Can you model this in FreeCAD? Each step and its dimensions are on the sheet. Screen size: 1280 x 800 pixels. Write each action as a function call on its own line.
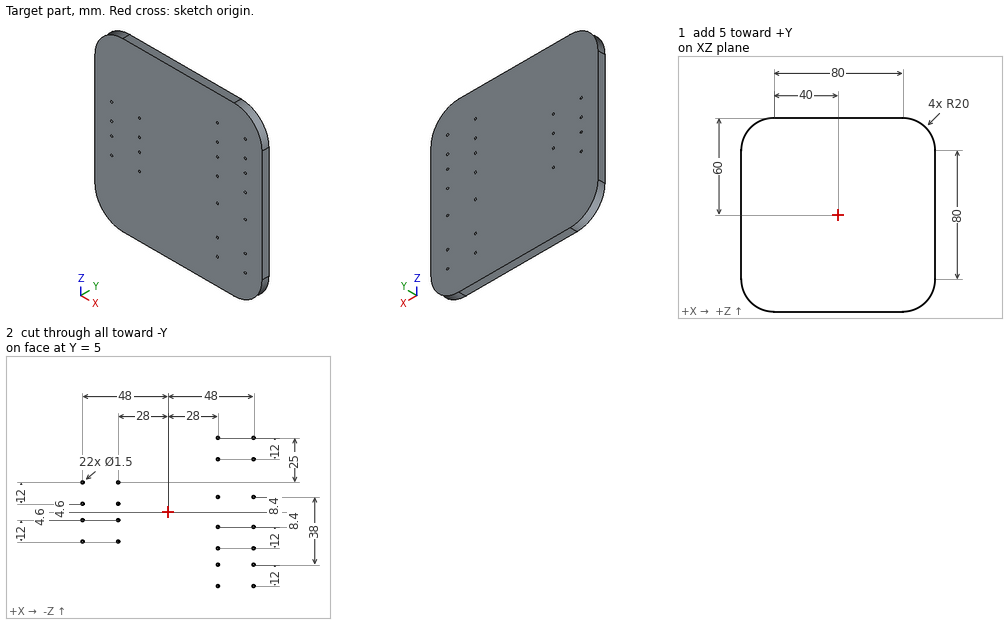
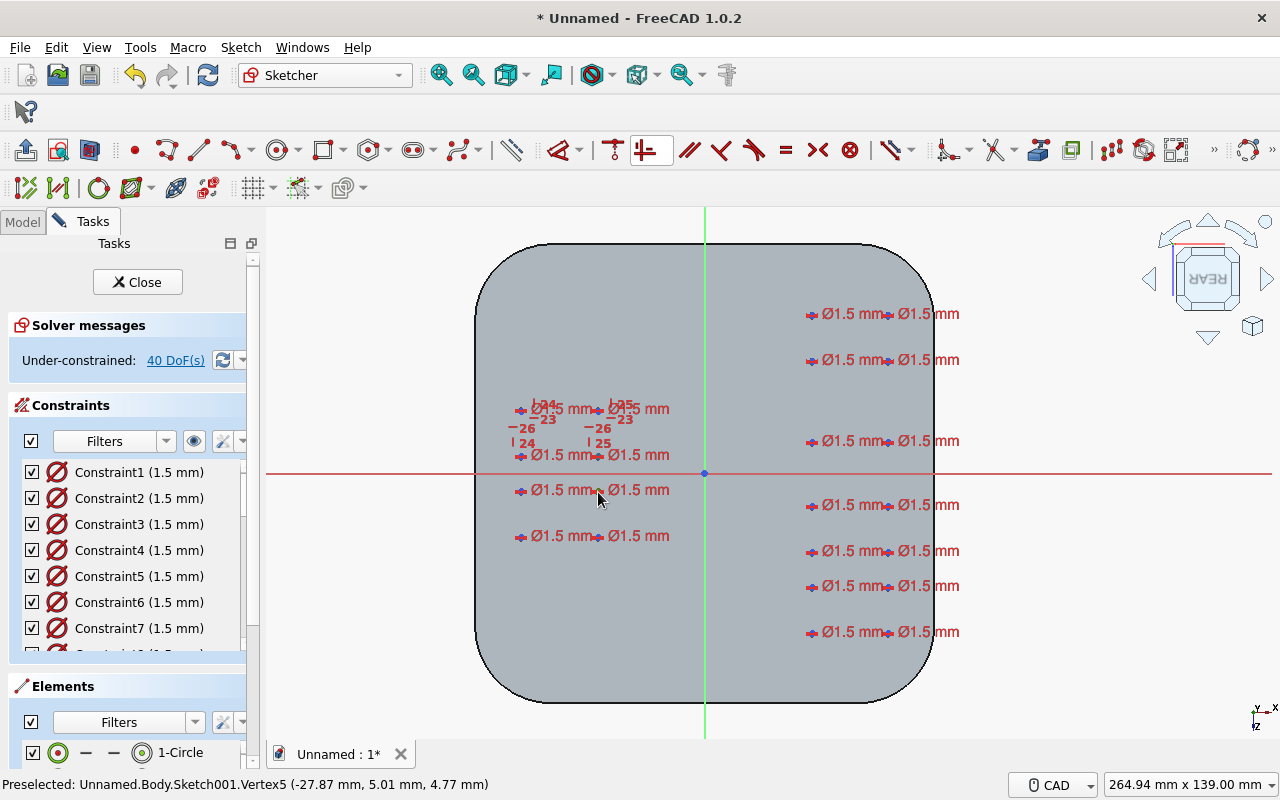
click(668, 150)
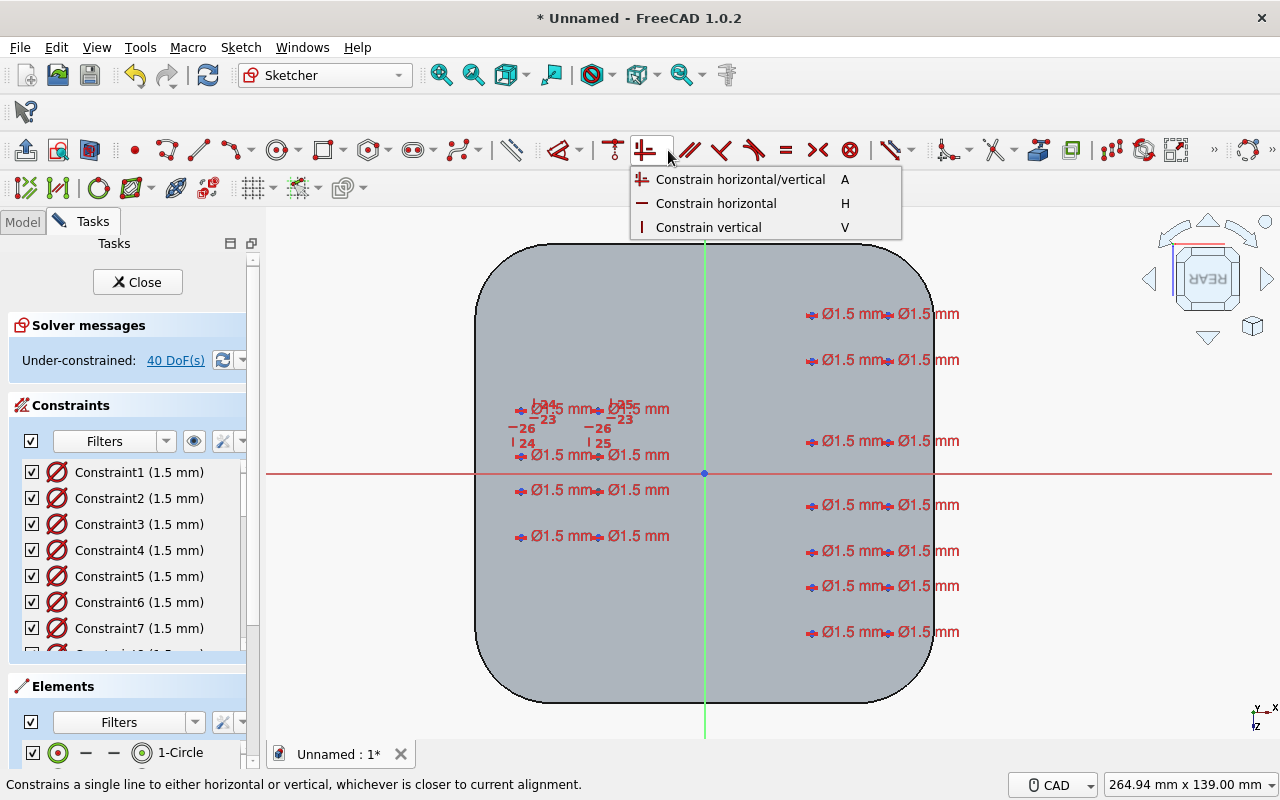
click(766, 227)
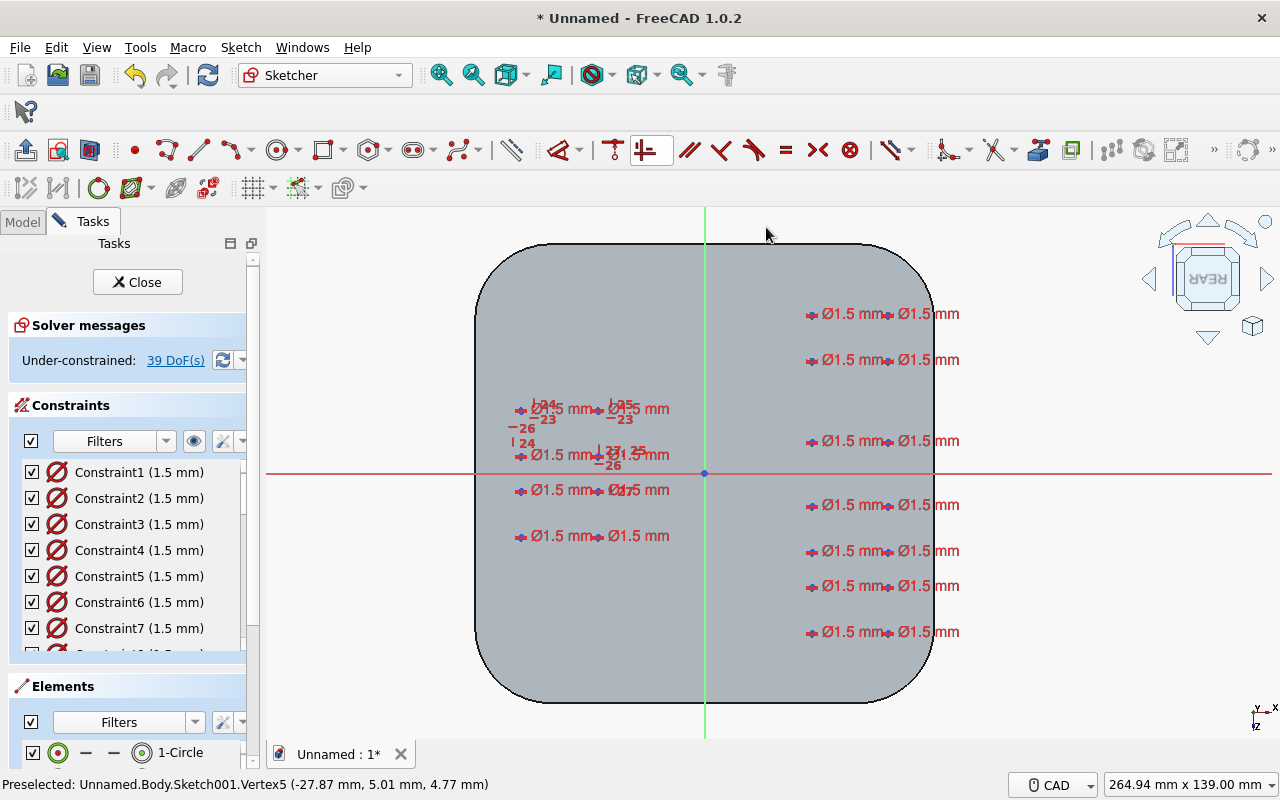
click(521, 457)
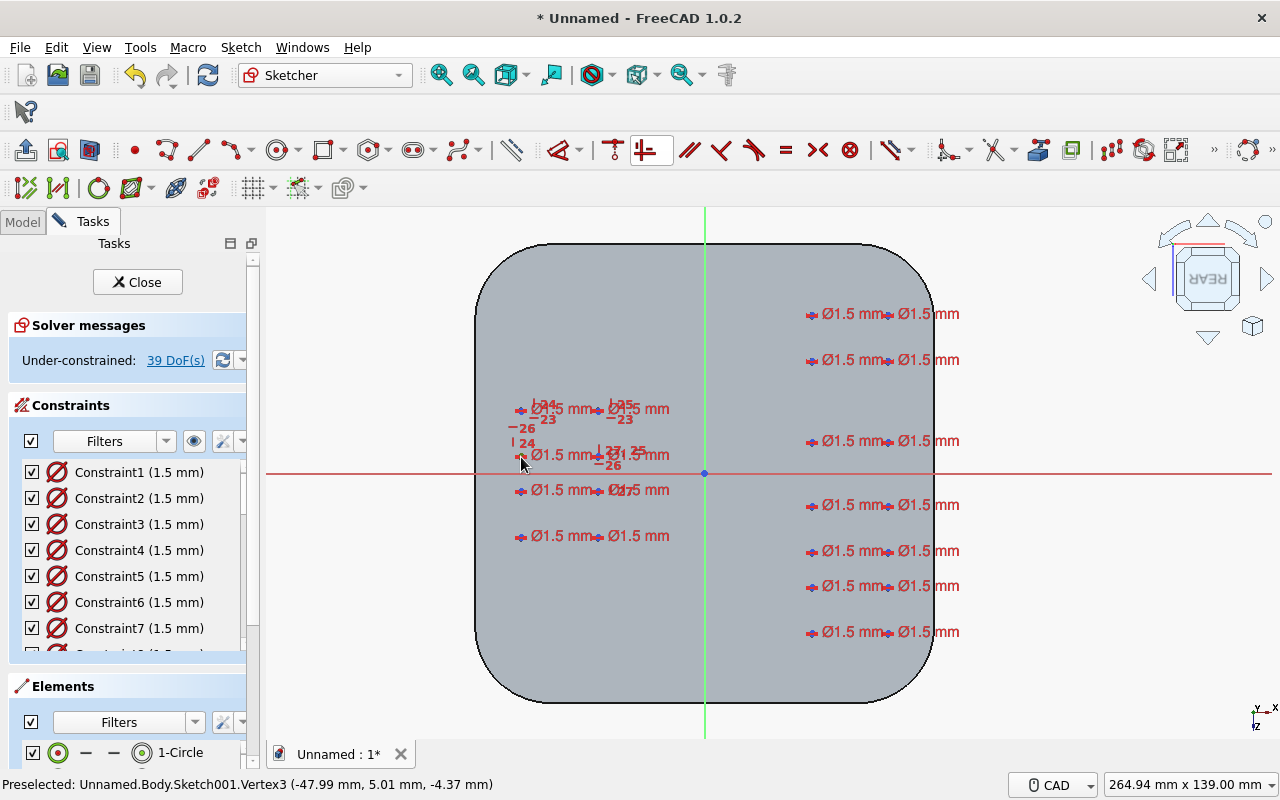
click(521, 492)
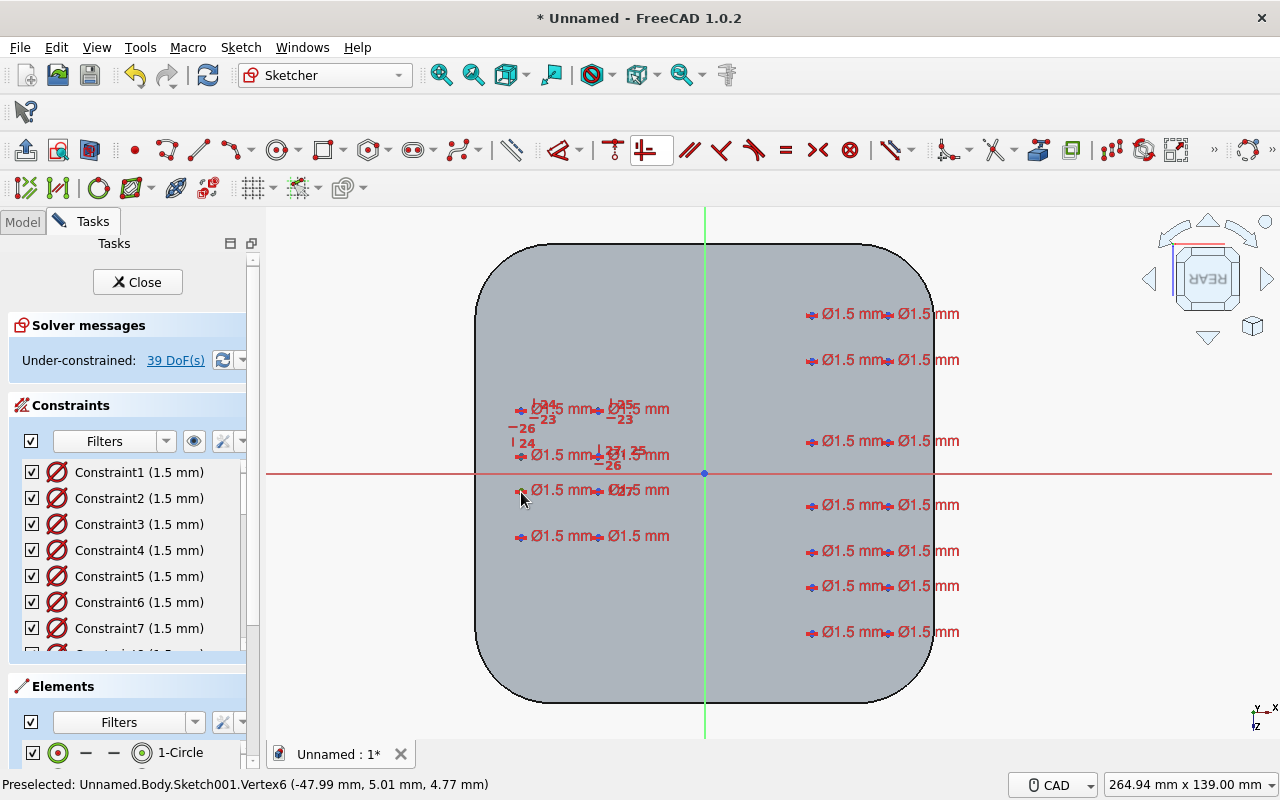
key(v)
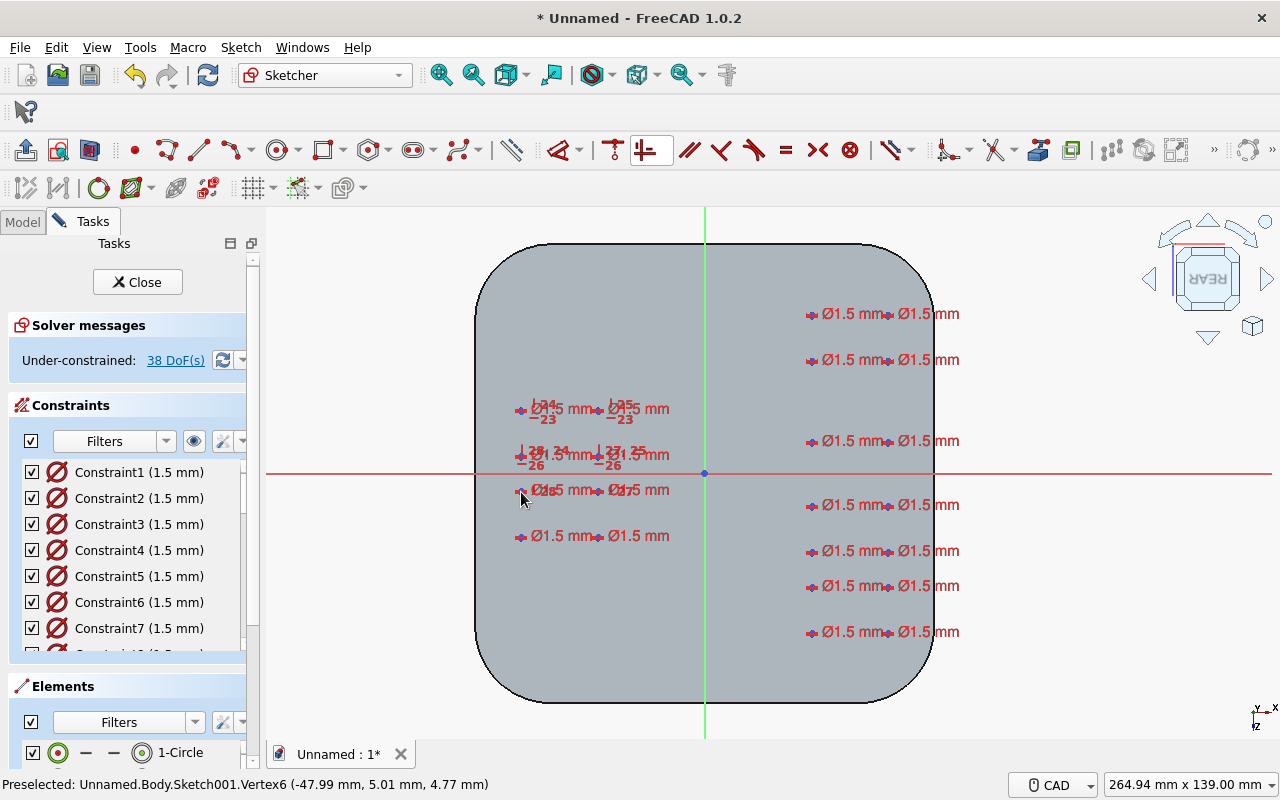
click(598, 492)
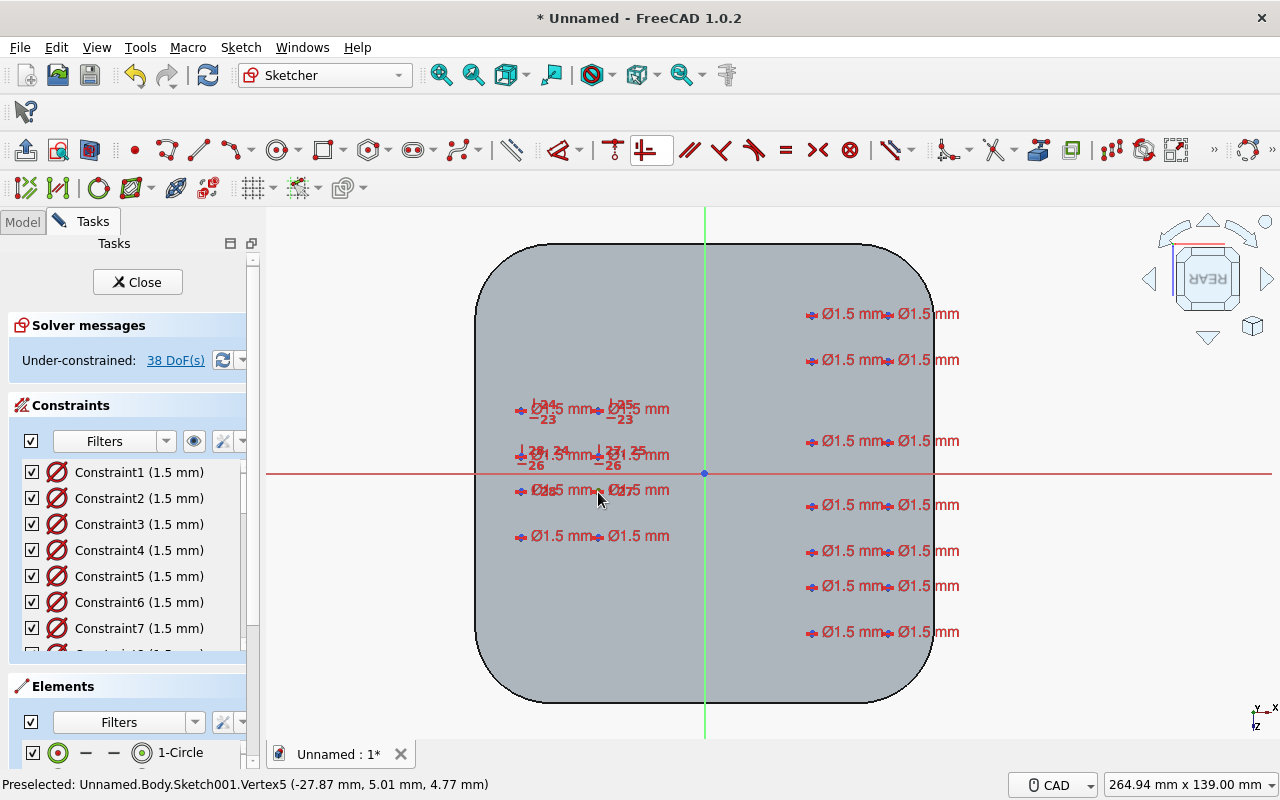
click(521, 492)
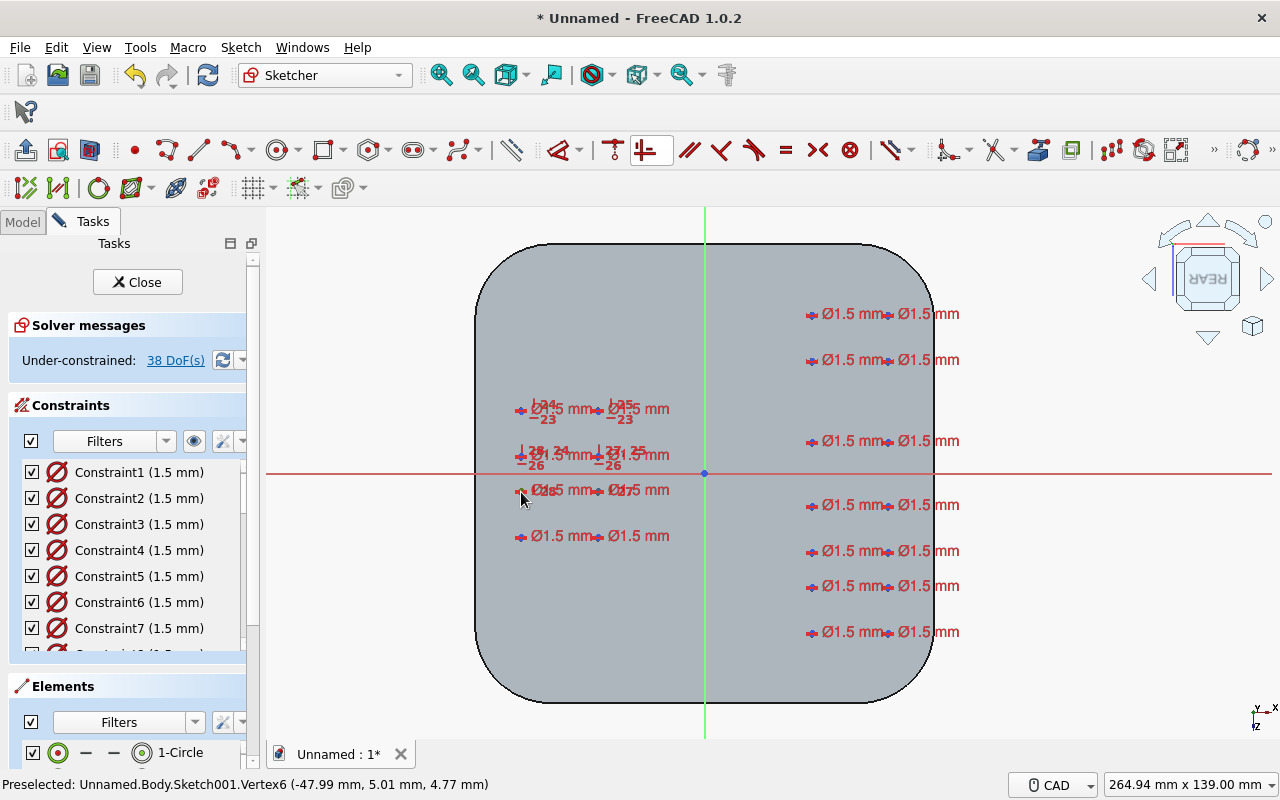
key(h)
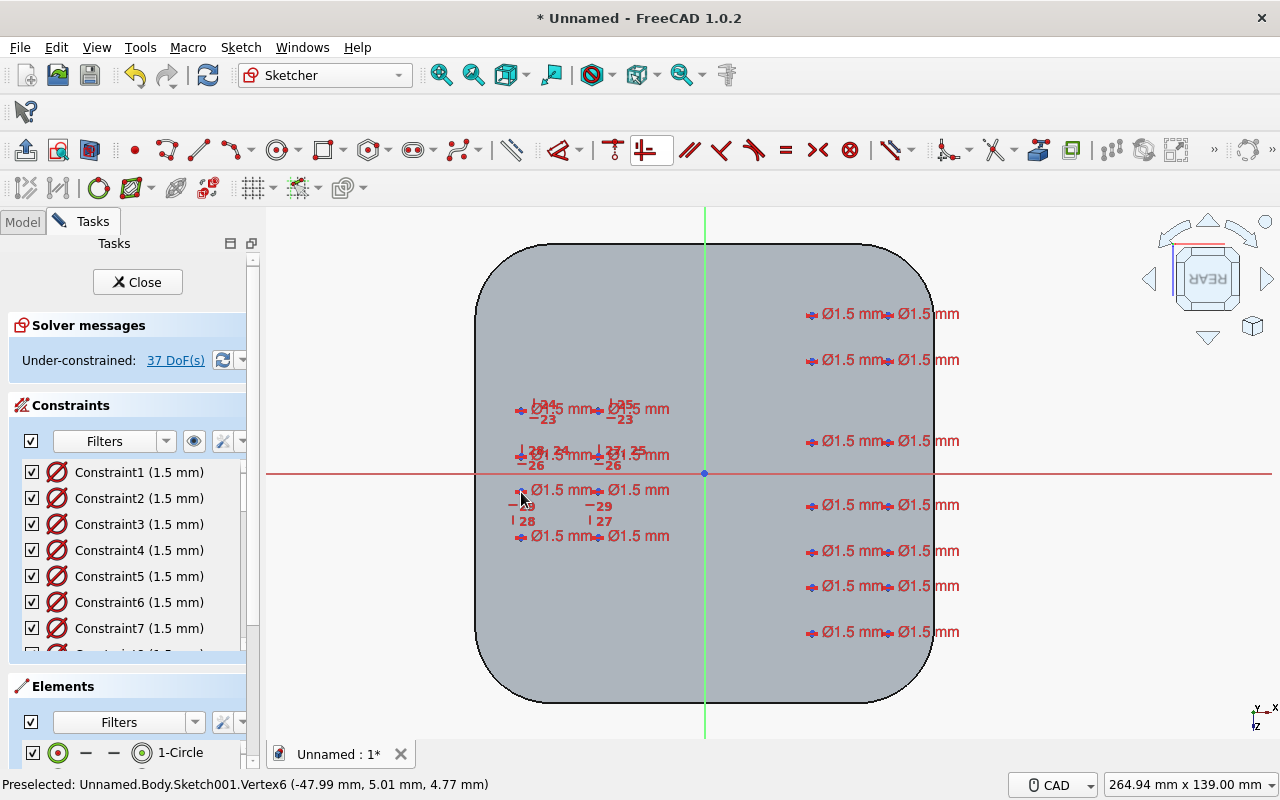
click(598, 492)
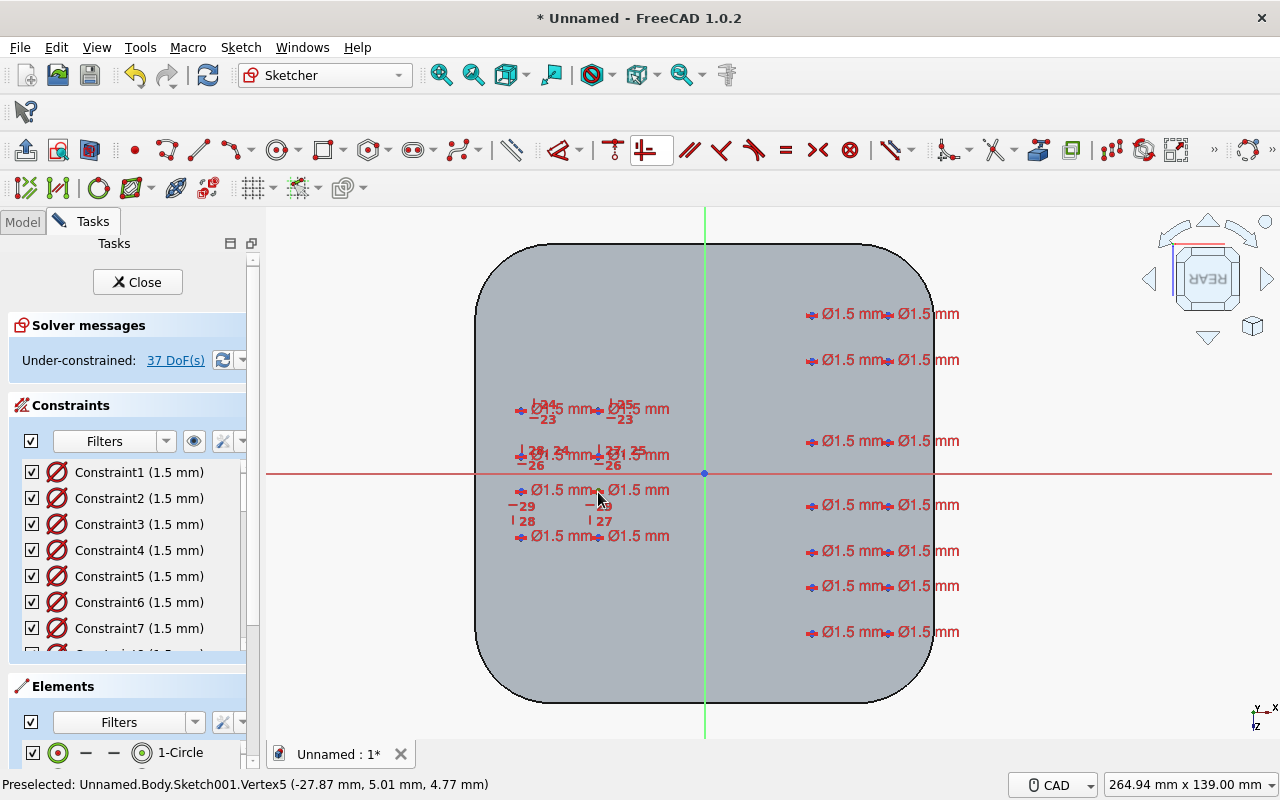
click(598, 538)